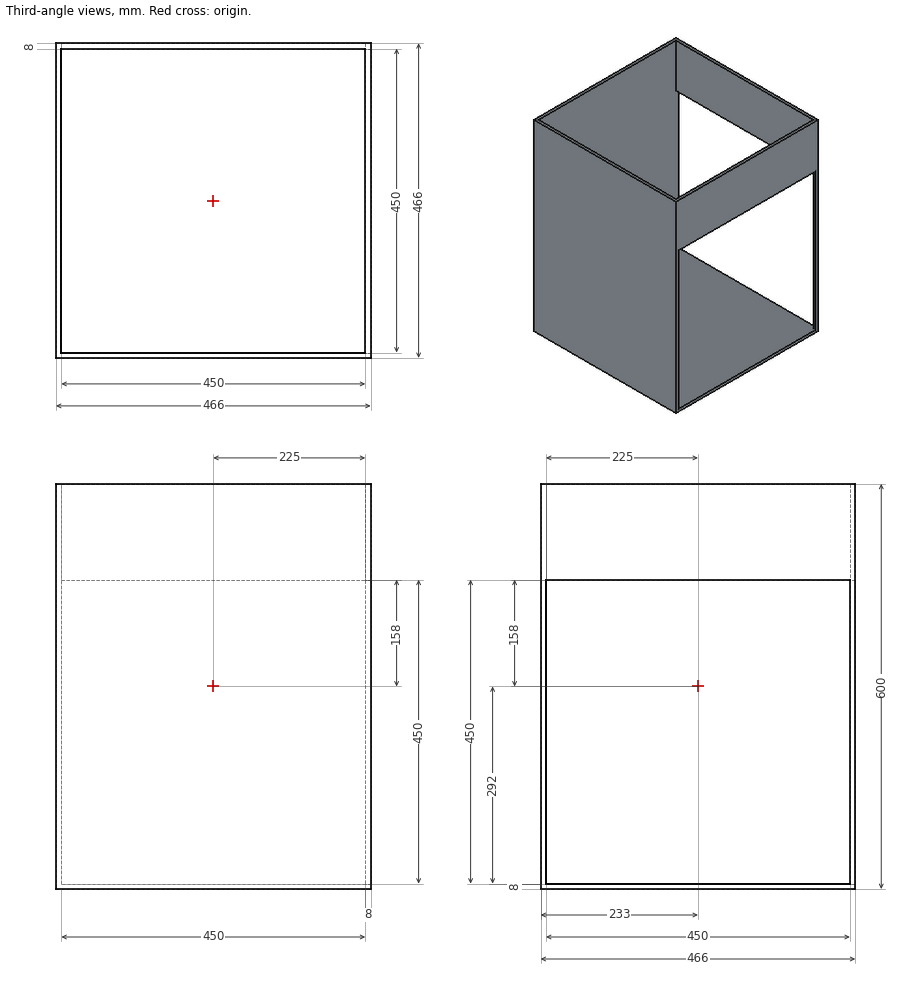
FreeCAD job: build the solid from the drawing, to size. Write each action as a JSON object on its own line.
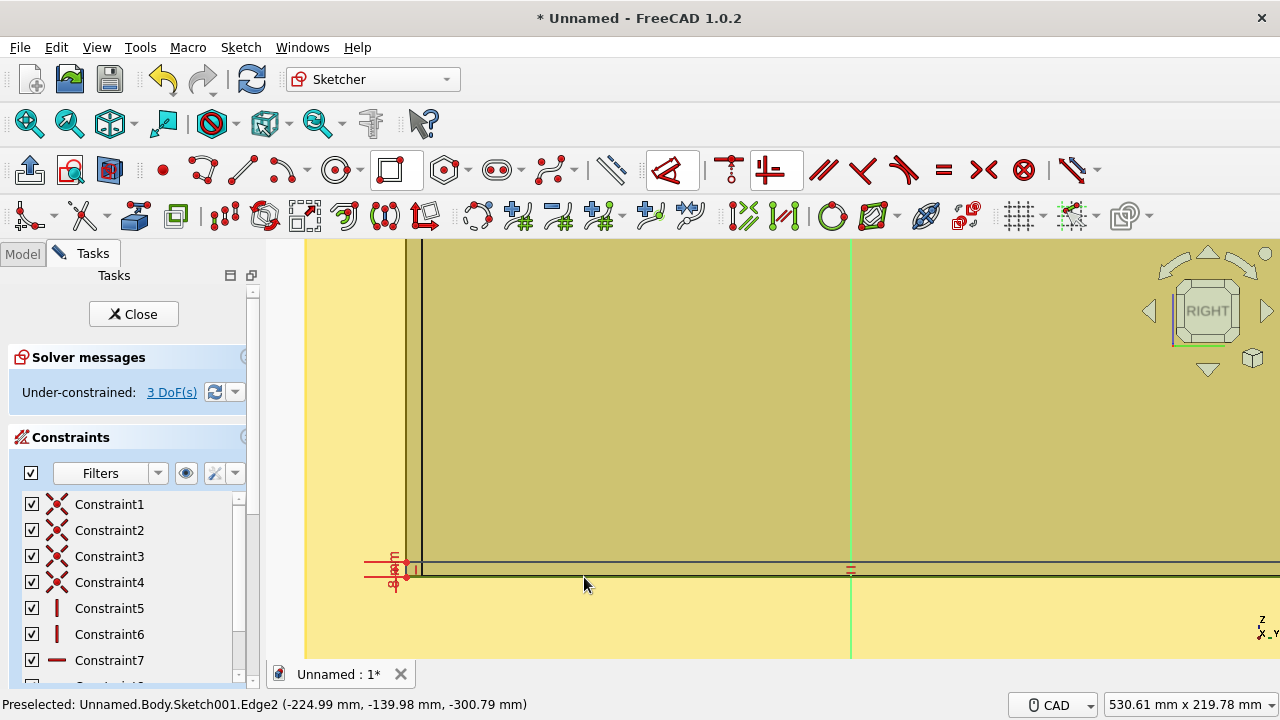
{"action": "left_click", "coordinate": [694, 170]}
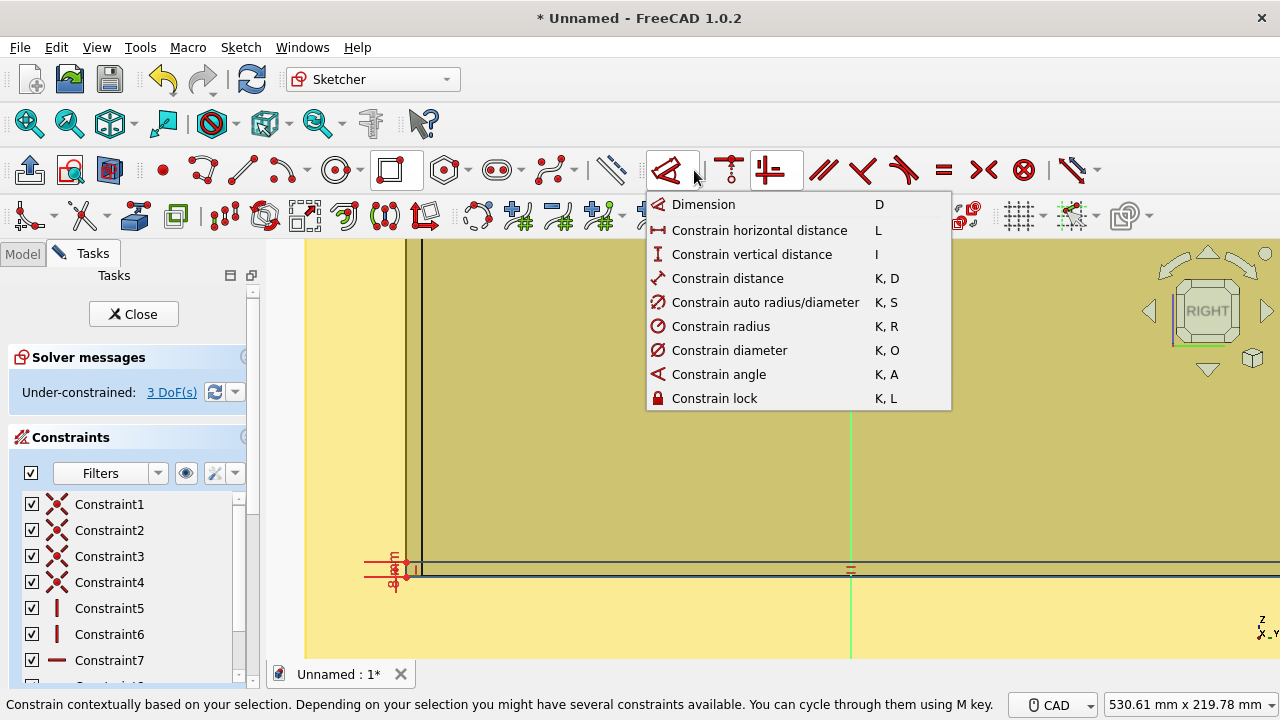
{"action": "left_click", "coordinate": [799, 230]}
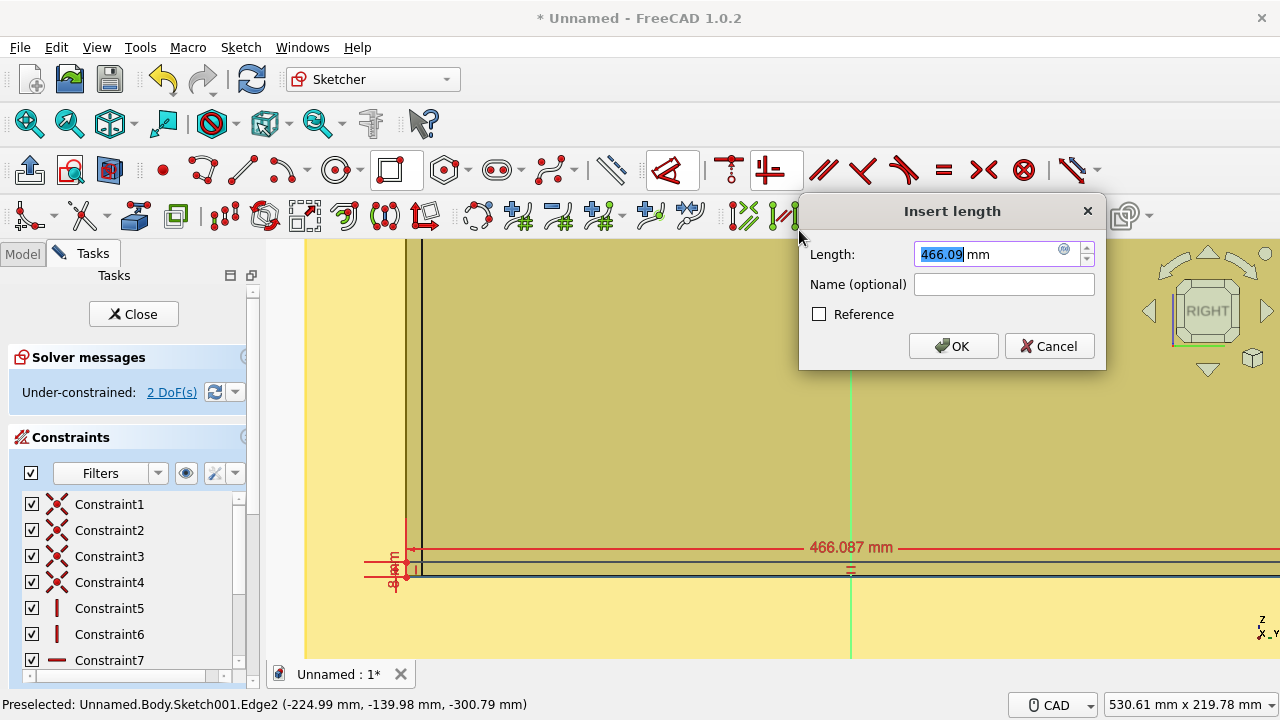
{"action": "type", "text": "466"}
{"action": "key", "text": "Return"}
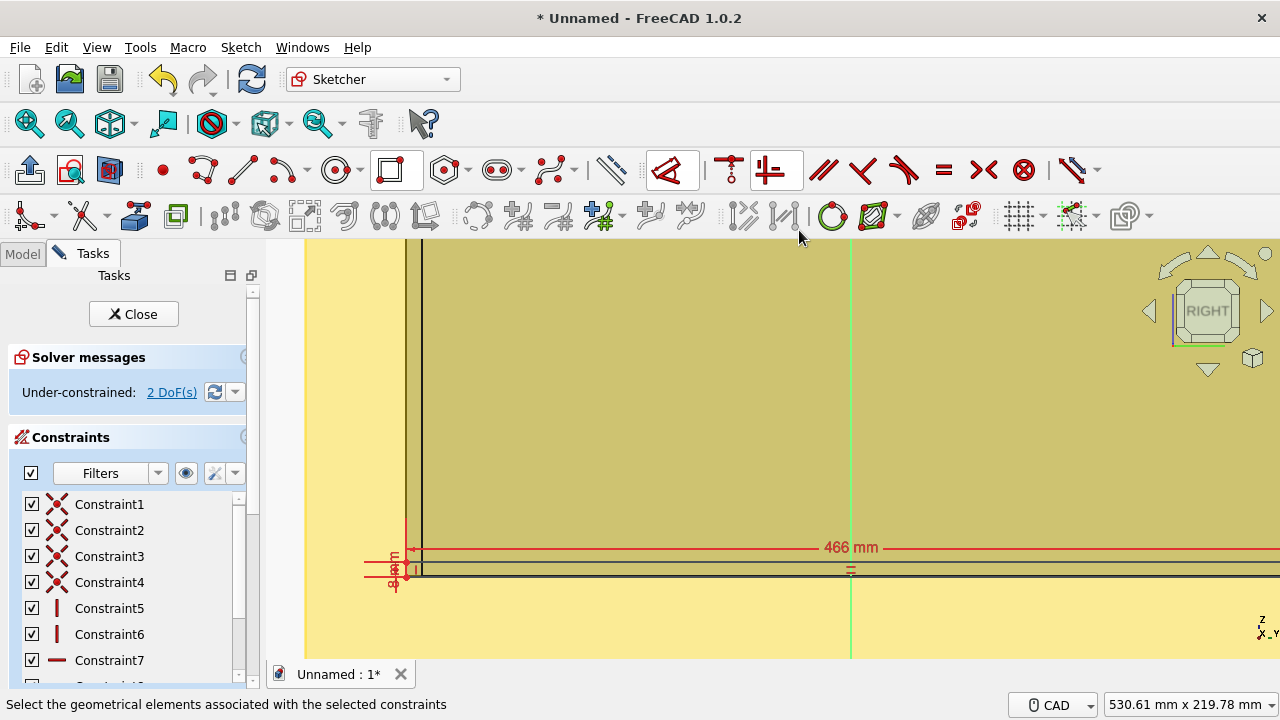
{"action": "left_click", "coordinate": [406, 562]}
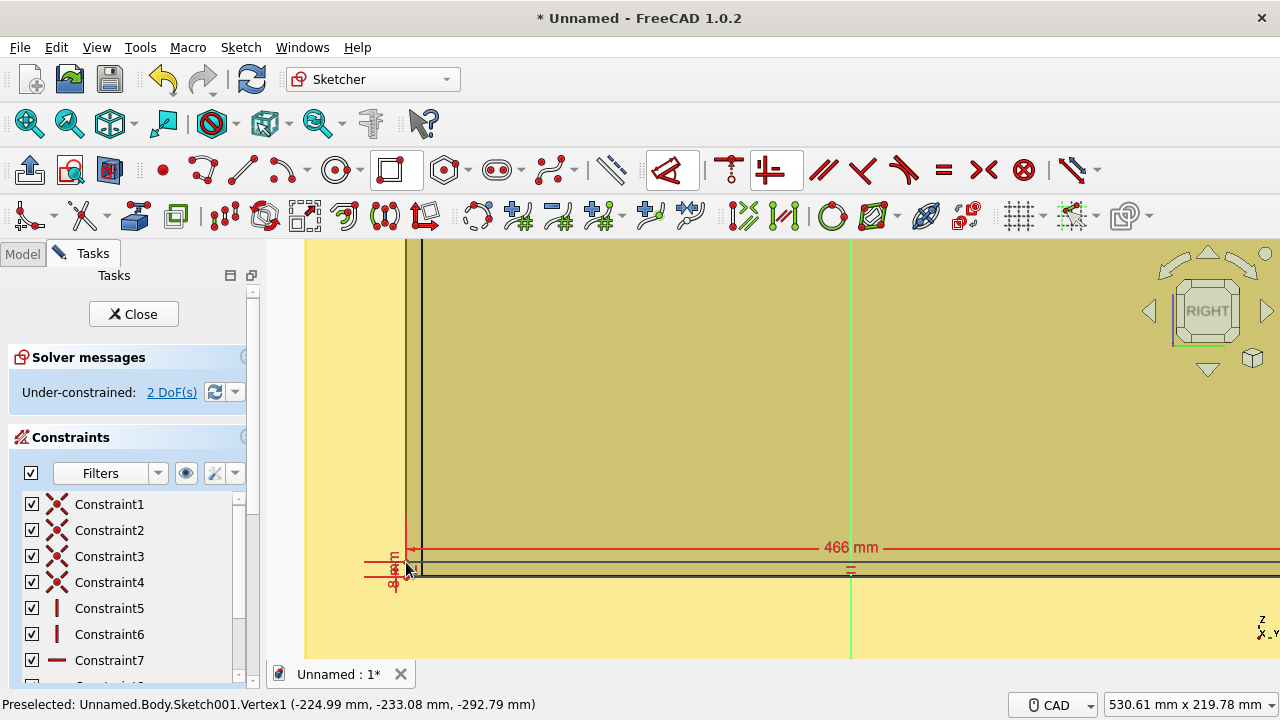
{"action": "left_click", "coordinate": [694, 170]}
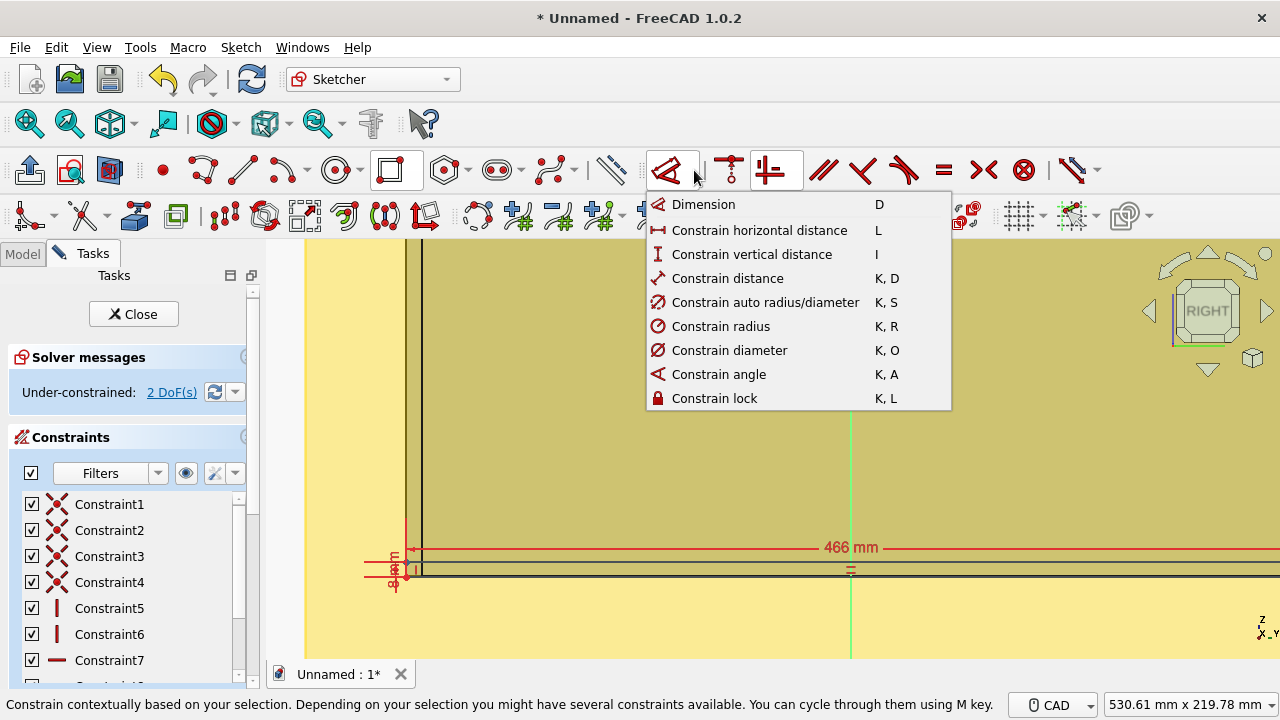
{"action": "left_click", "coordinate": [799, 230]}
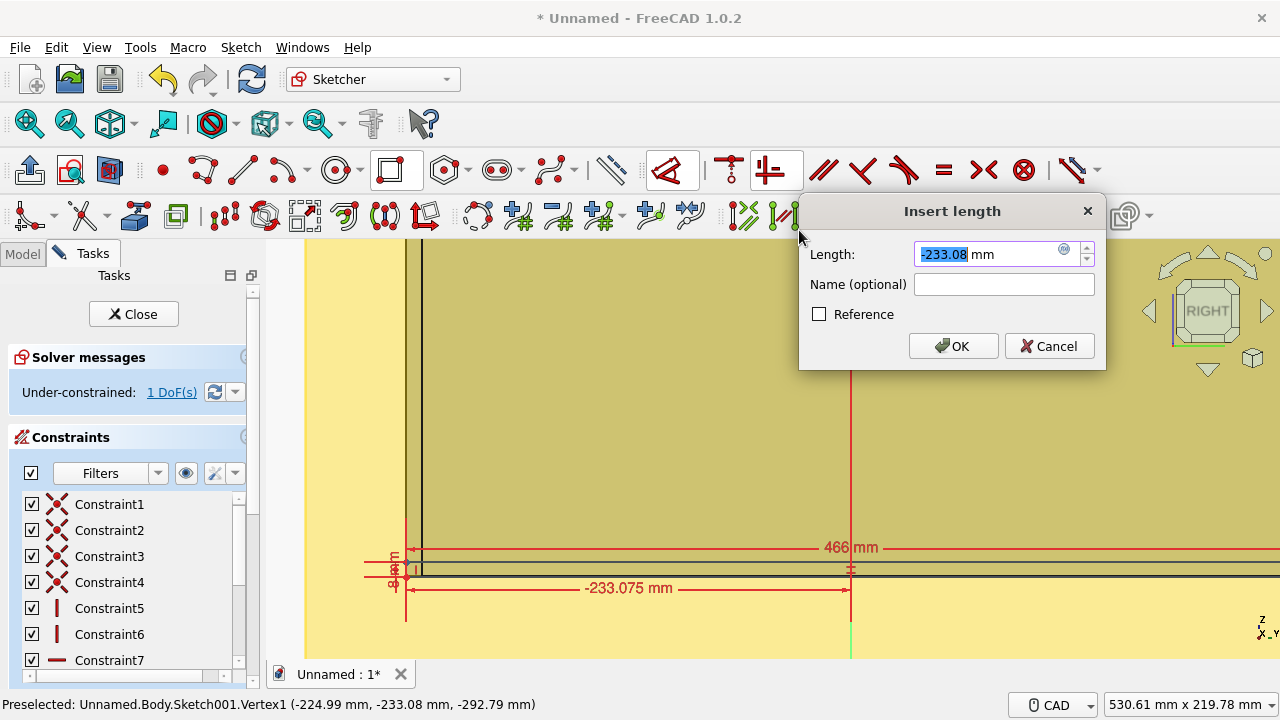
{"action": "type", "text": "-233"}
{"action": "key", "text": "Return"}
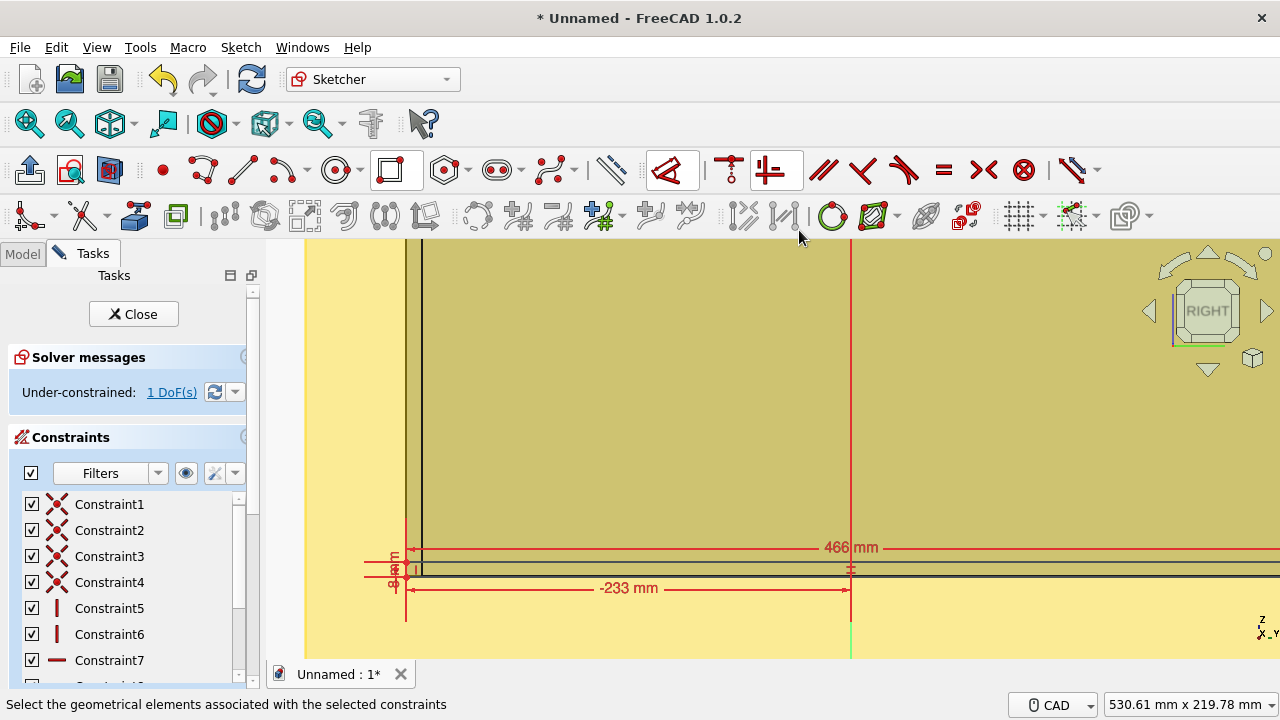
{"action": "left_click", "coordinate": [406, 562]}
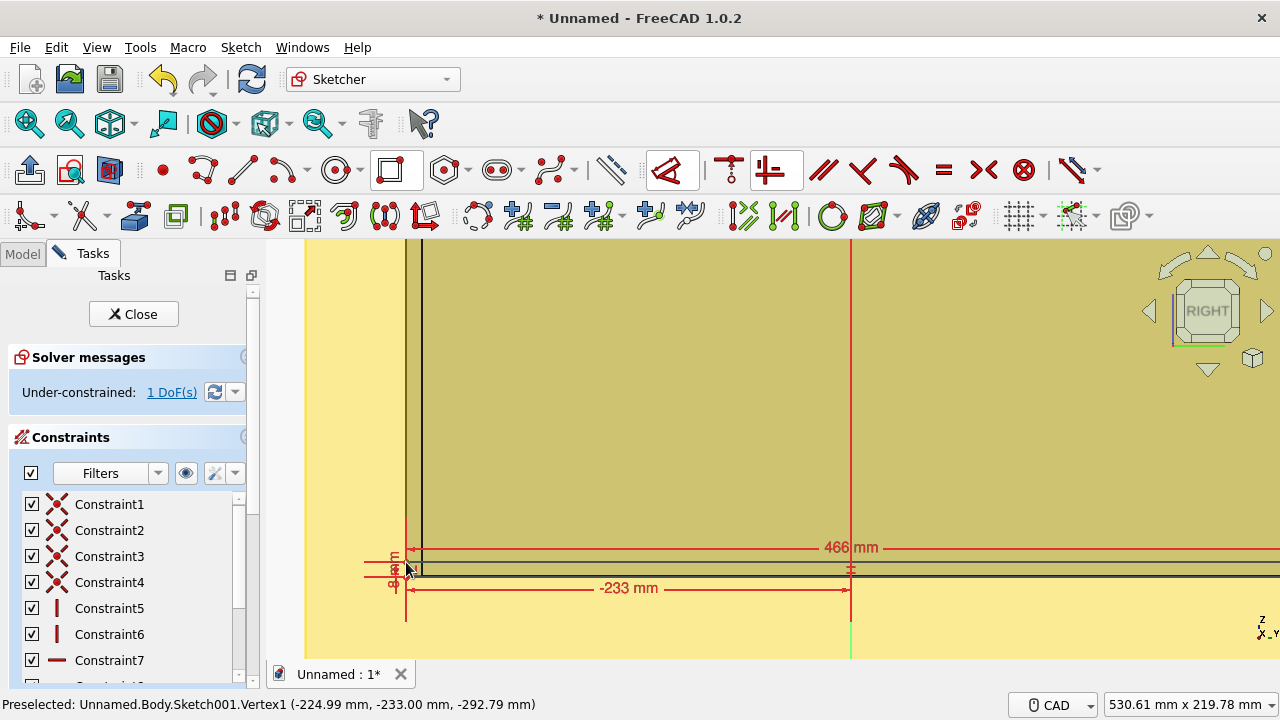
{"action": "left_click", "coordinate": [694, 170]}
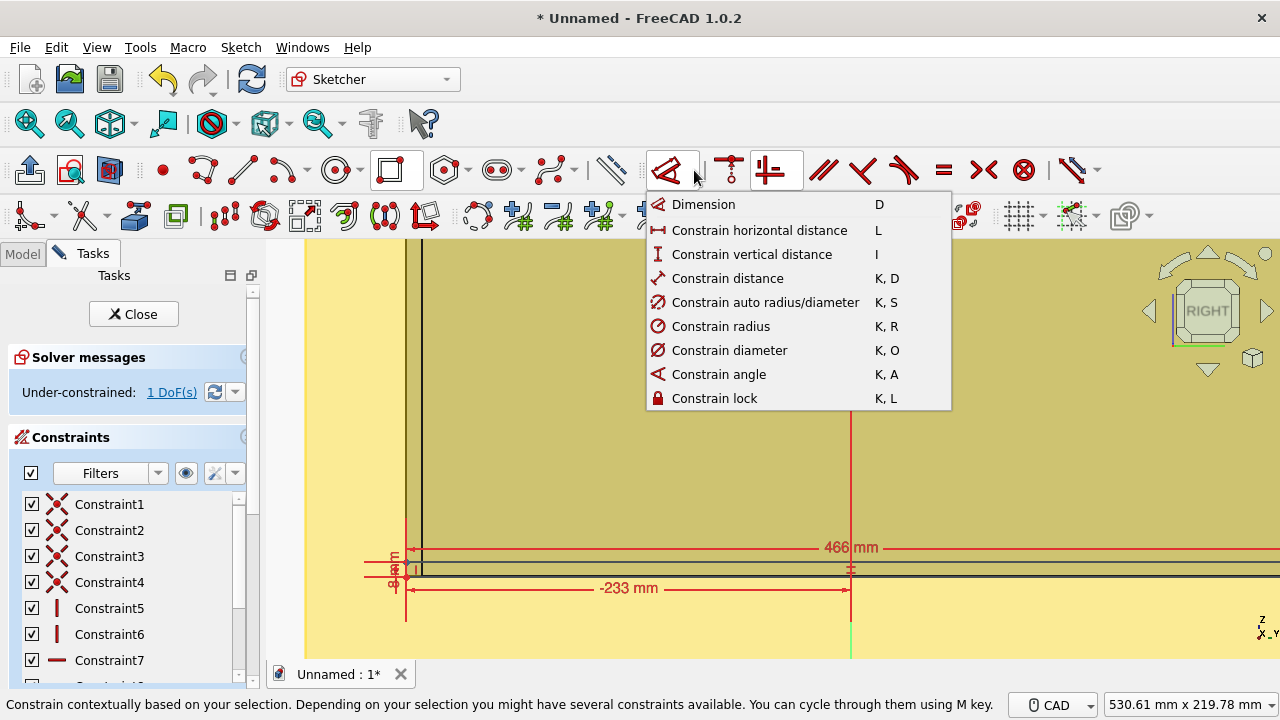
{"action": "left_click", "coordinate": [799, 254]}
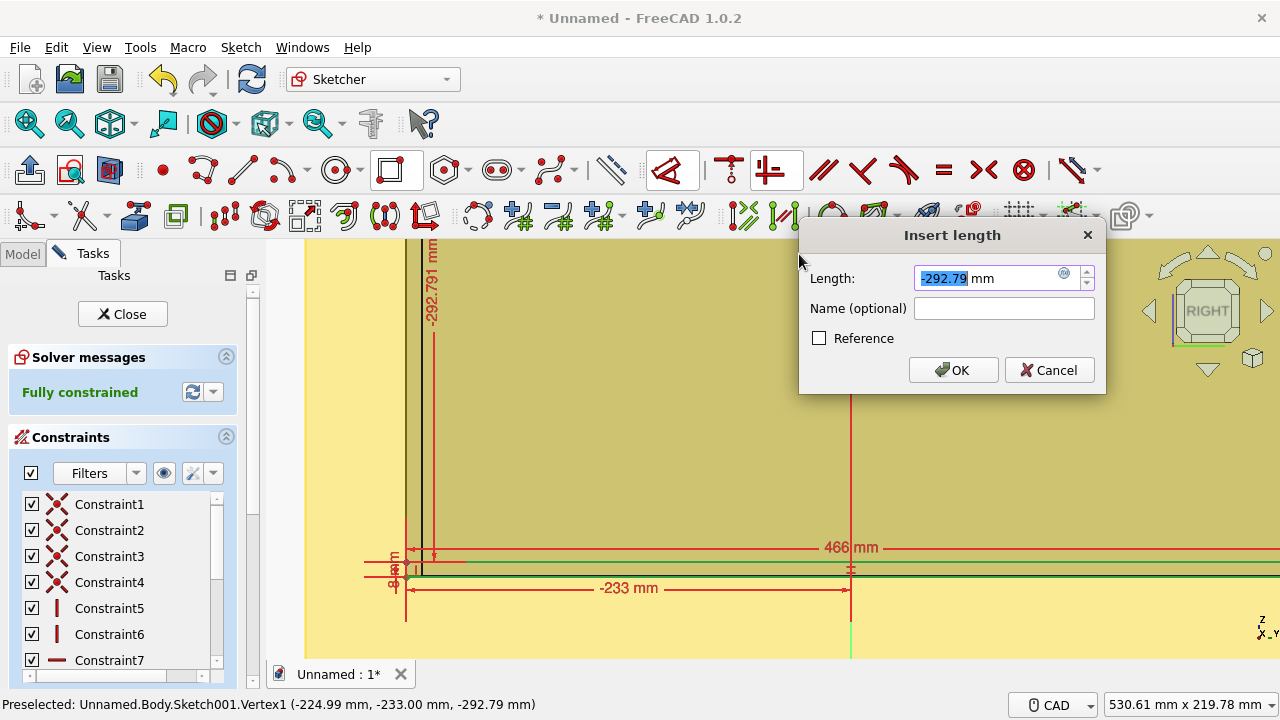
{"action": "type", "text": "-292"}
{"action": "key", "text": "Return"}